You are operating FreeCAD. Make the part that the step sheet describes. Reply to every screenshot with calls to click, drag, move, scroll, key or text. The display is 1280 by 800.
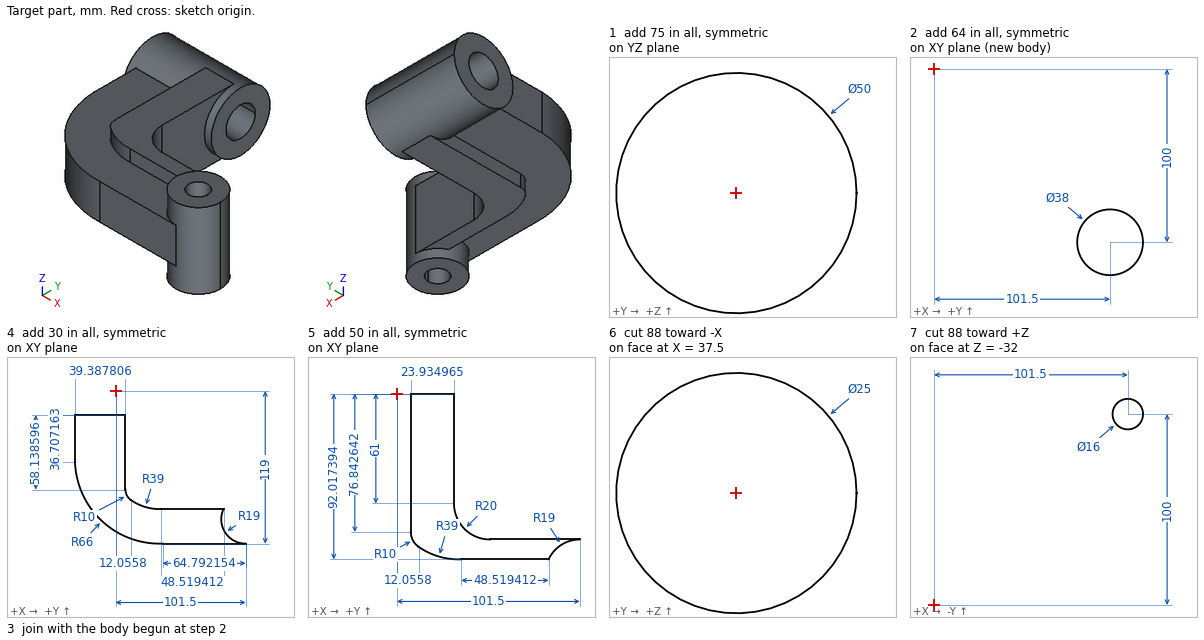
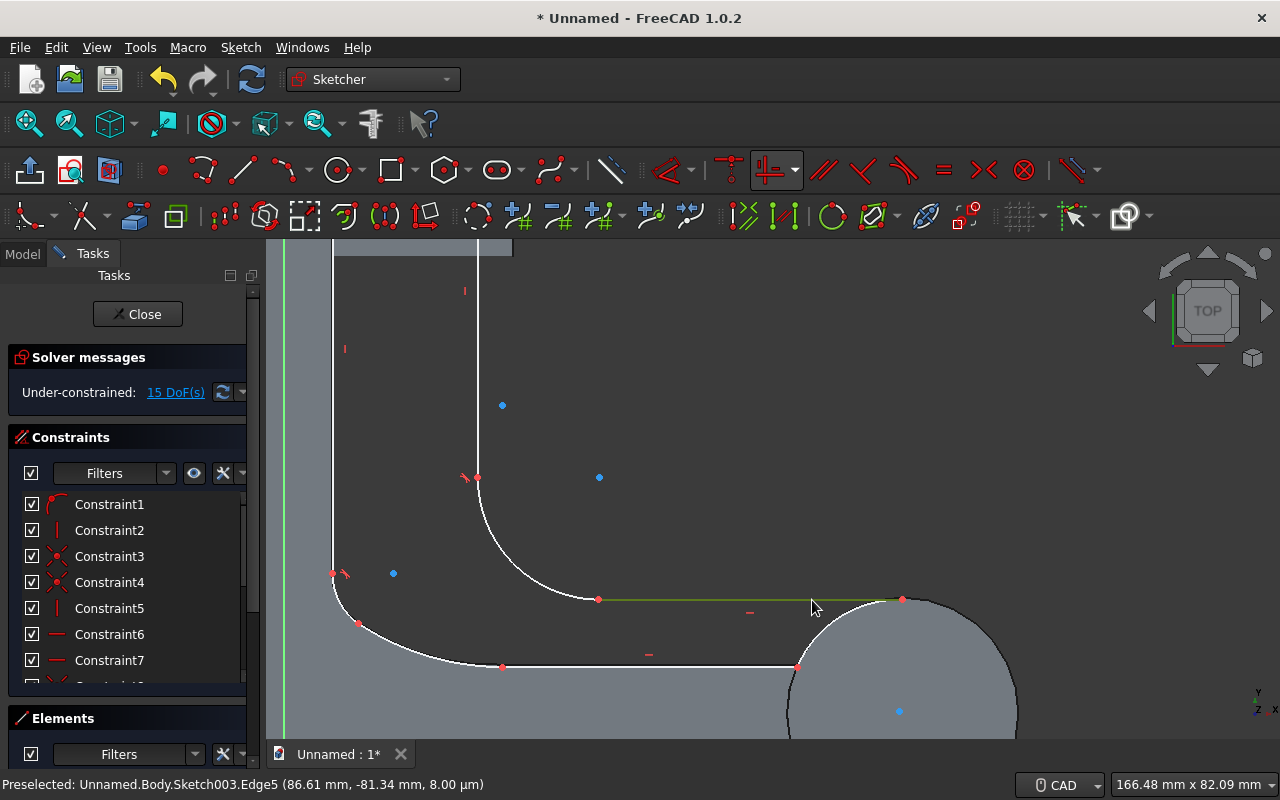
click(819, 634)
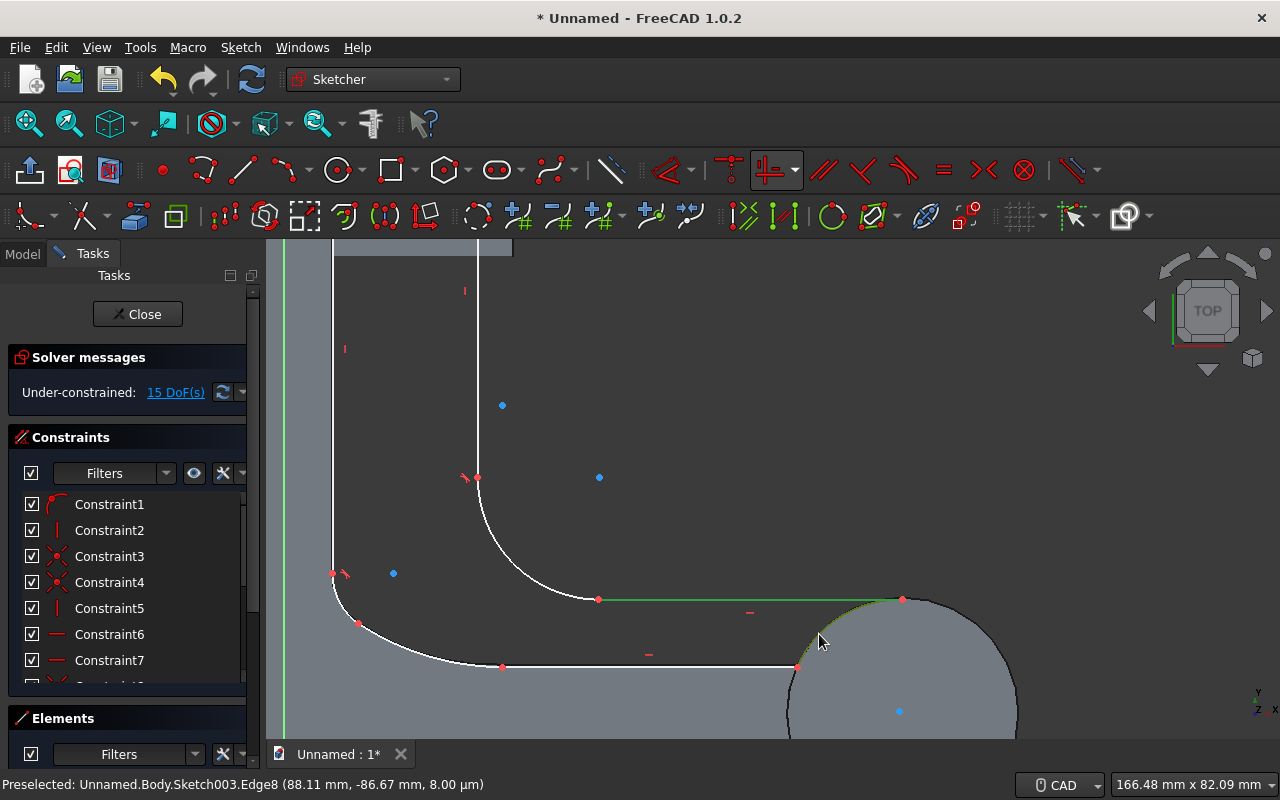
click(904, 170)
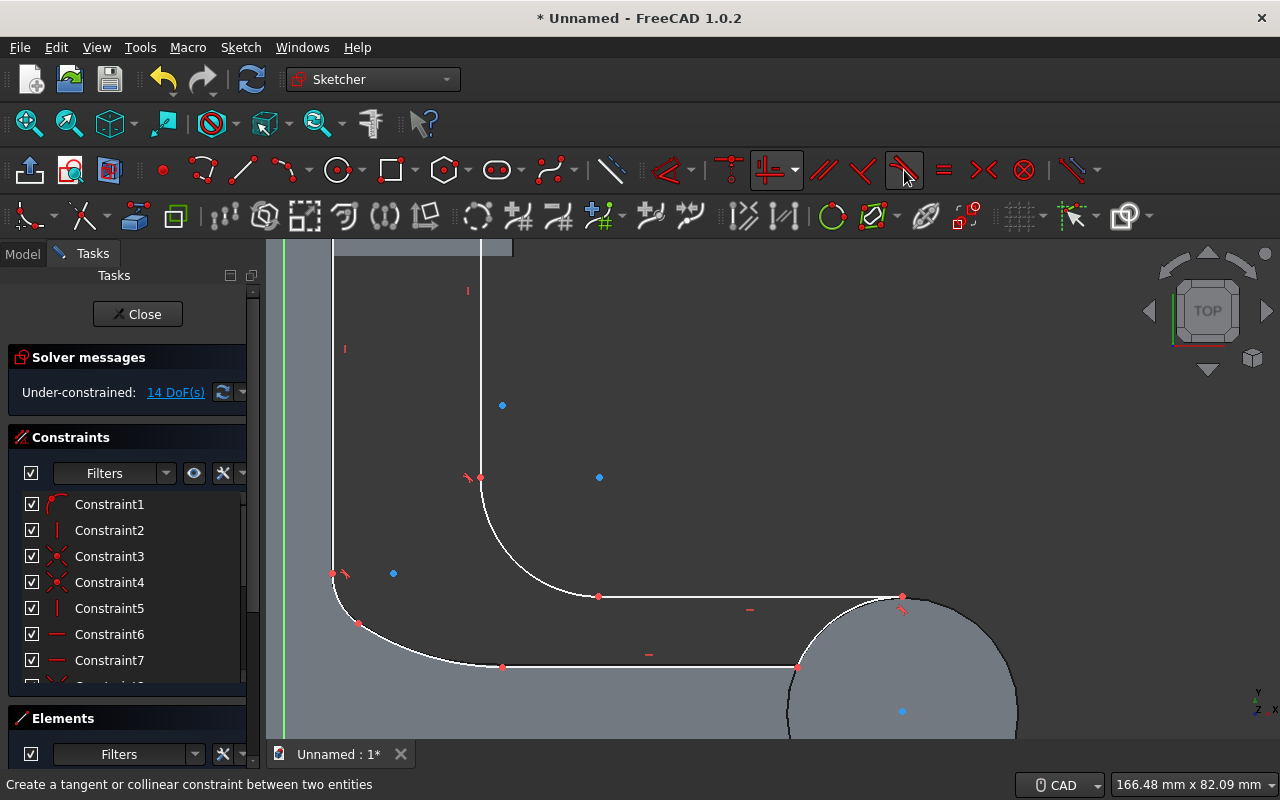
click(812, 597)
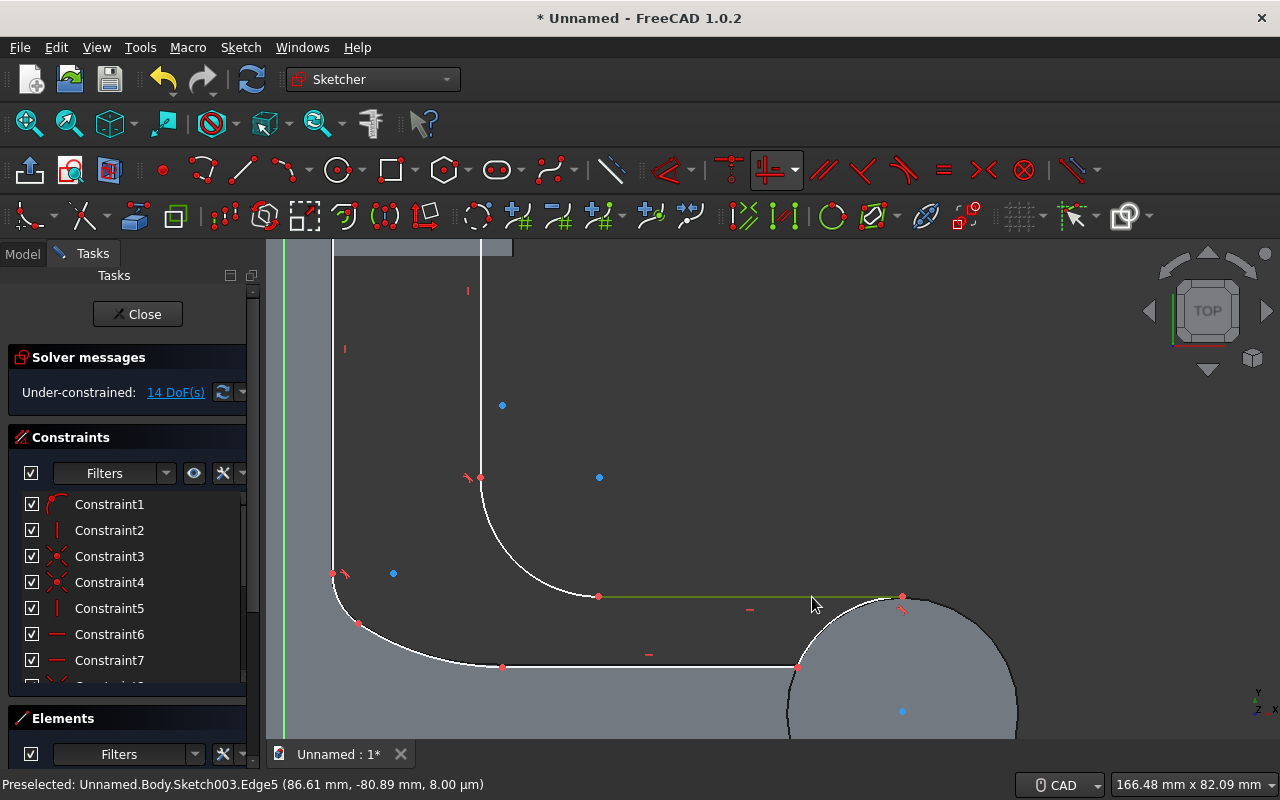
click(493, 531)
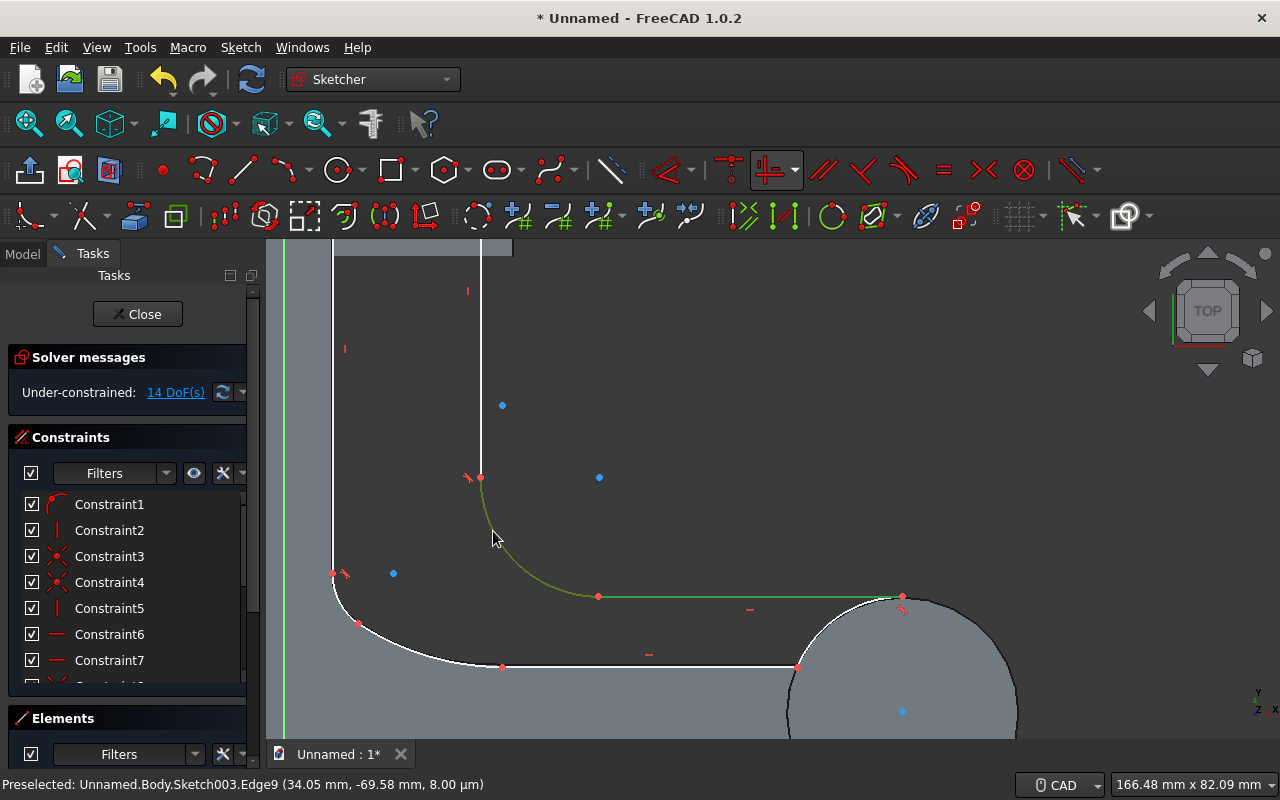
click(904, 170)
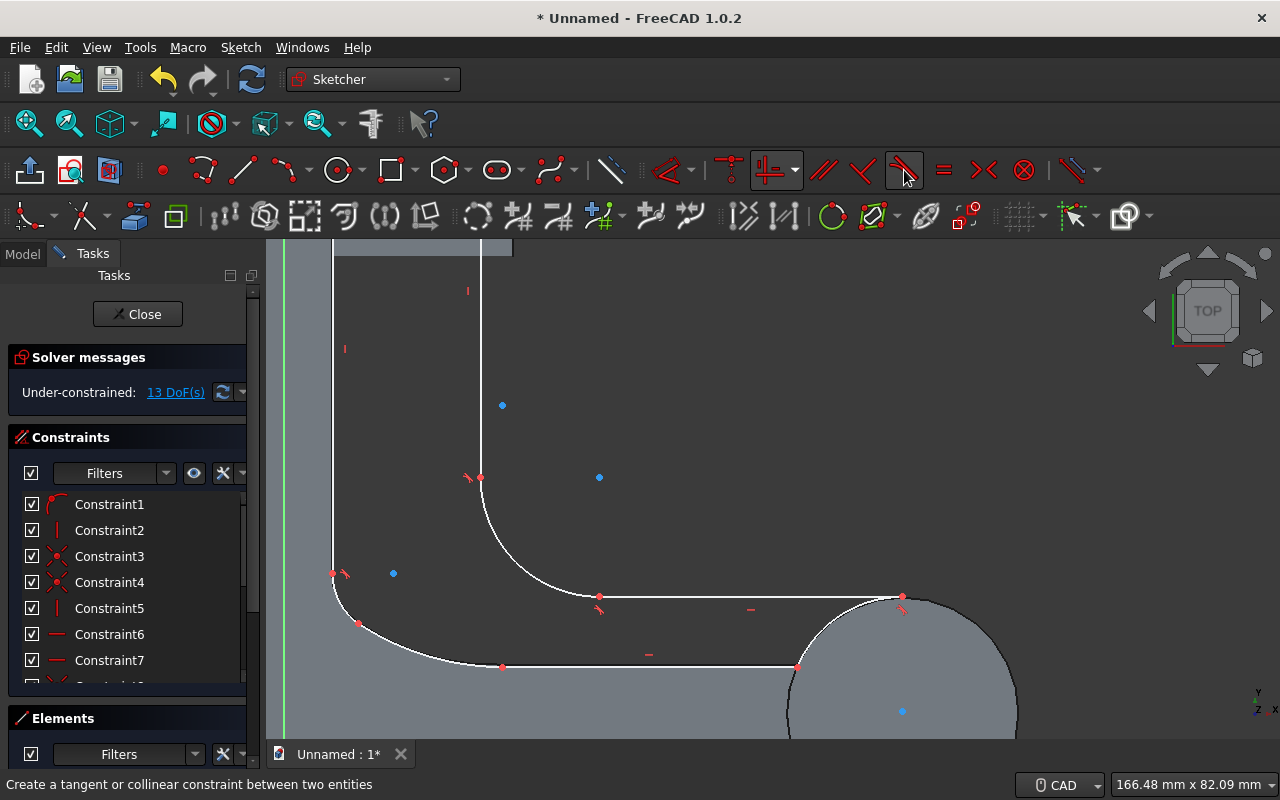
click(335, 591)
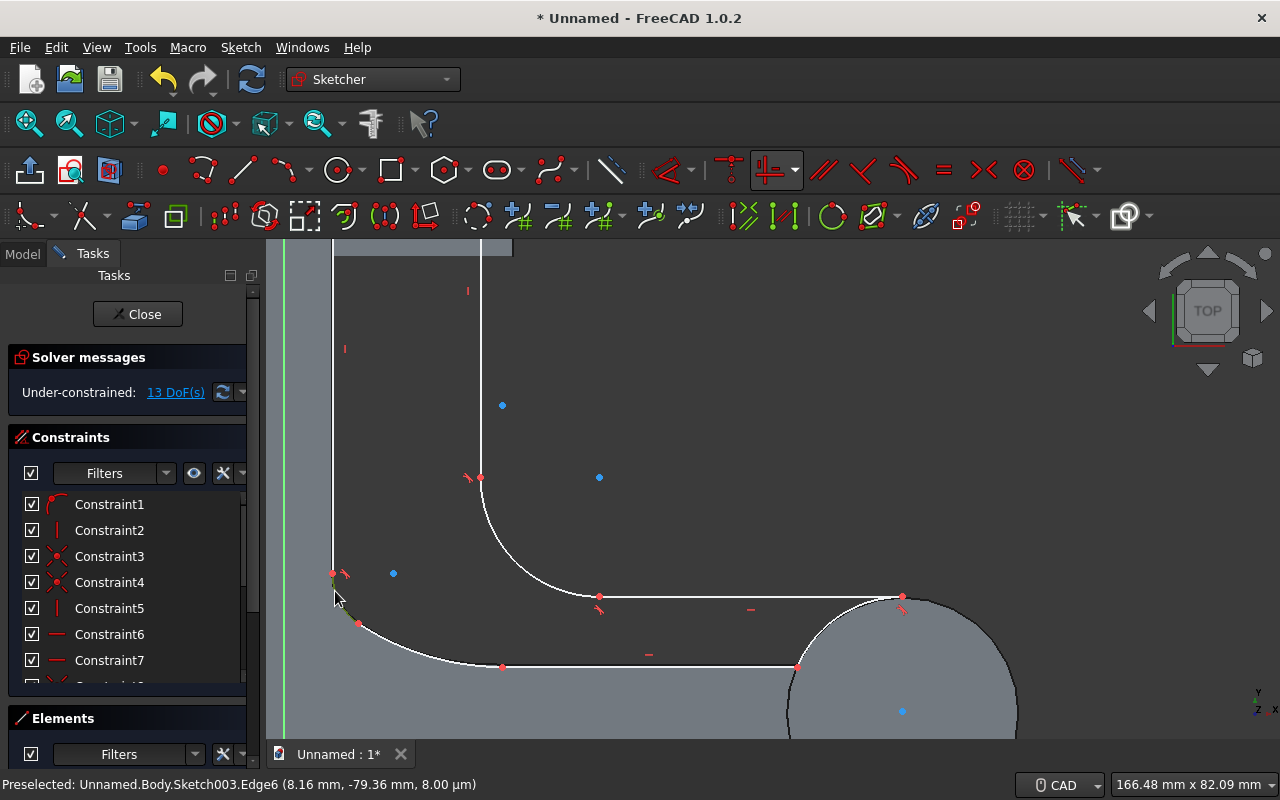
click(398, 645)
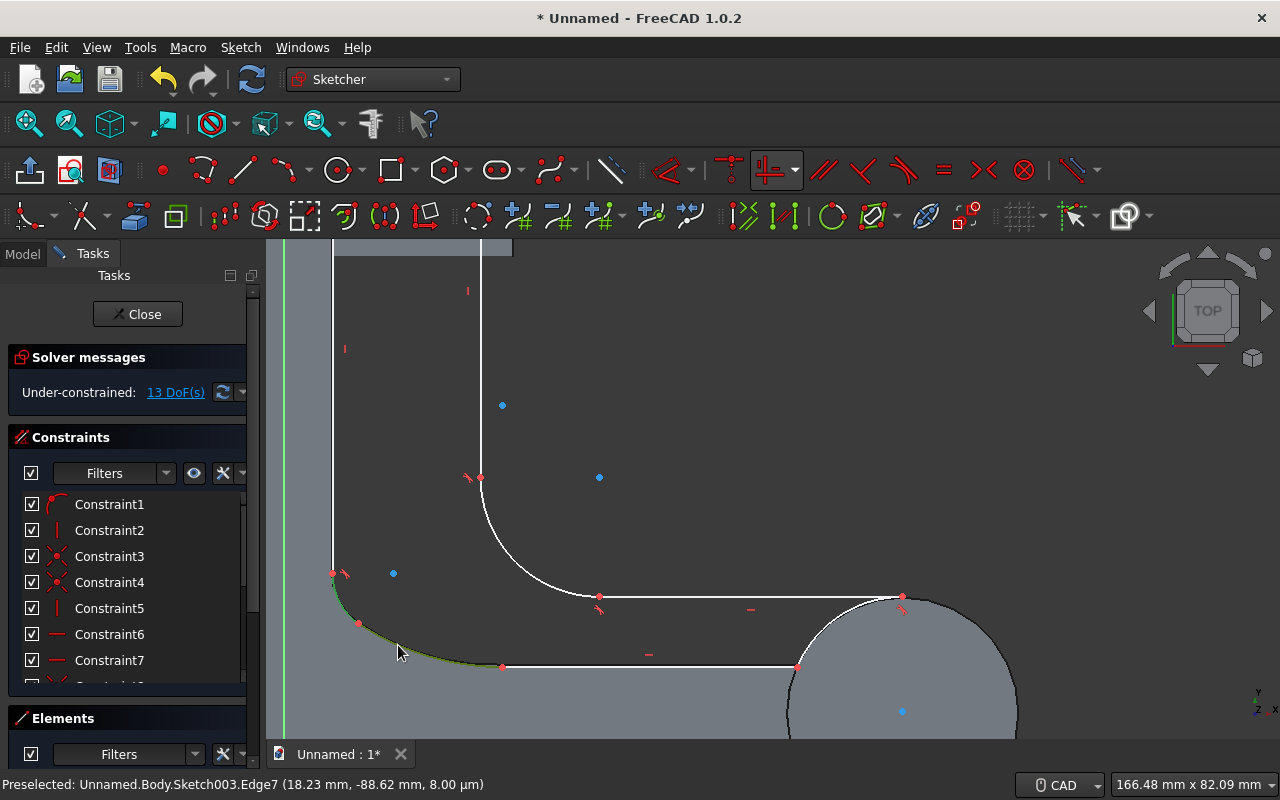
click(904, 170)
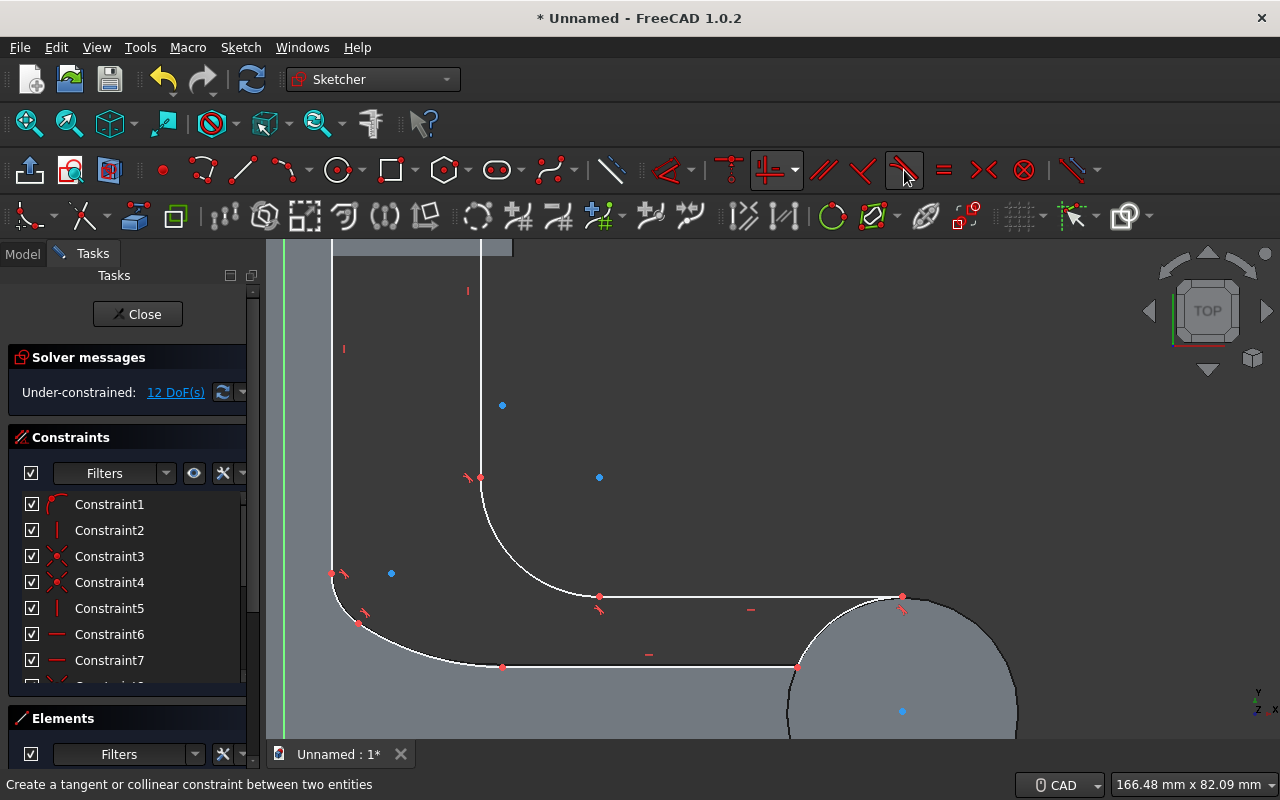
scroll(839, 616, down, 3)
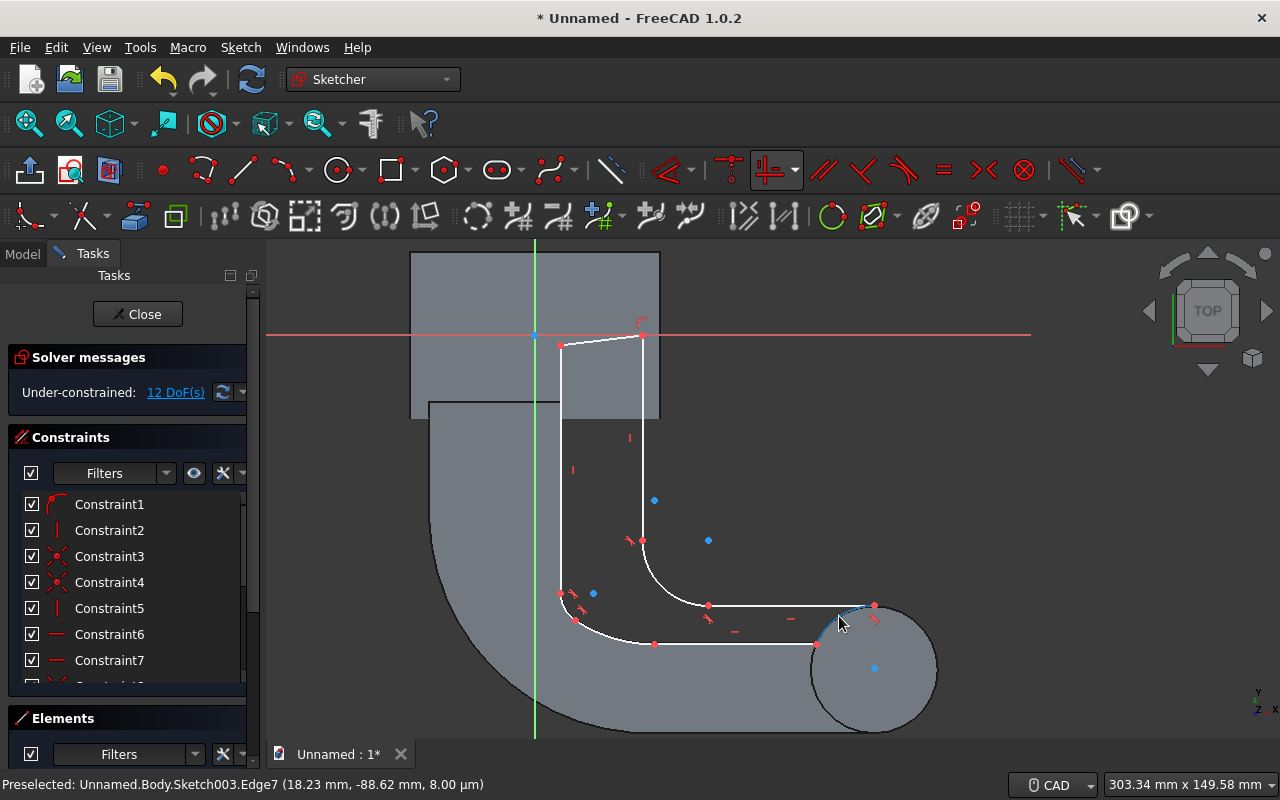
scroll(585, 342, up, 4)